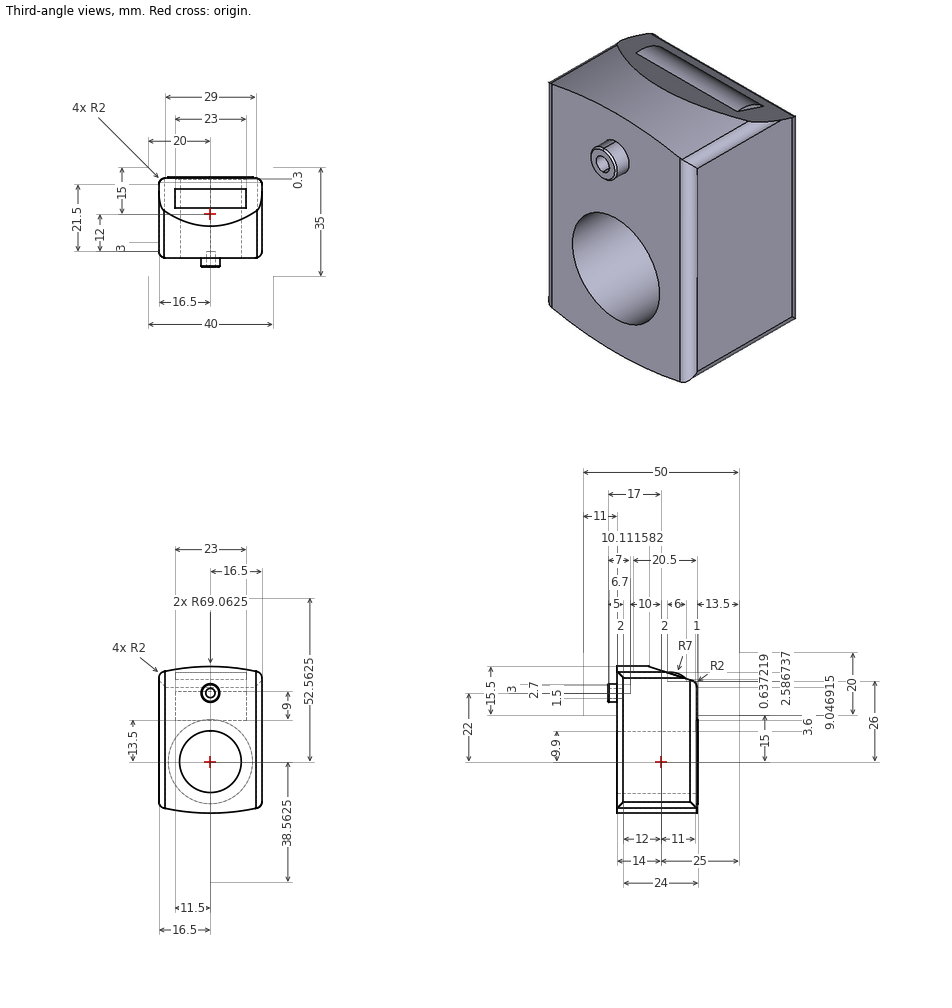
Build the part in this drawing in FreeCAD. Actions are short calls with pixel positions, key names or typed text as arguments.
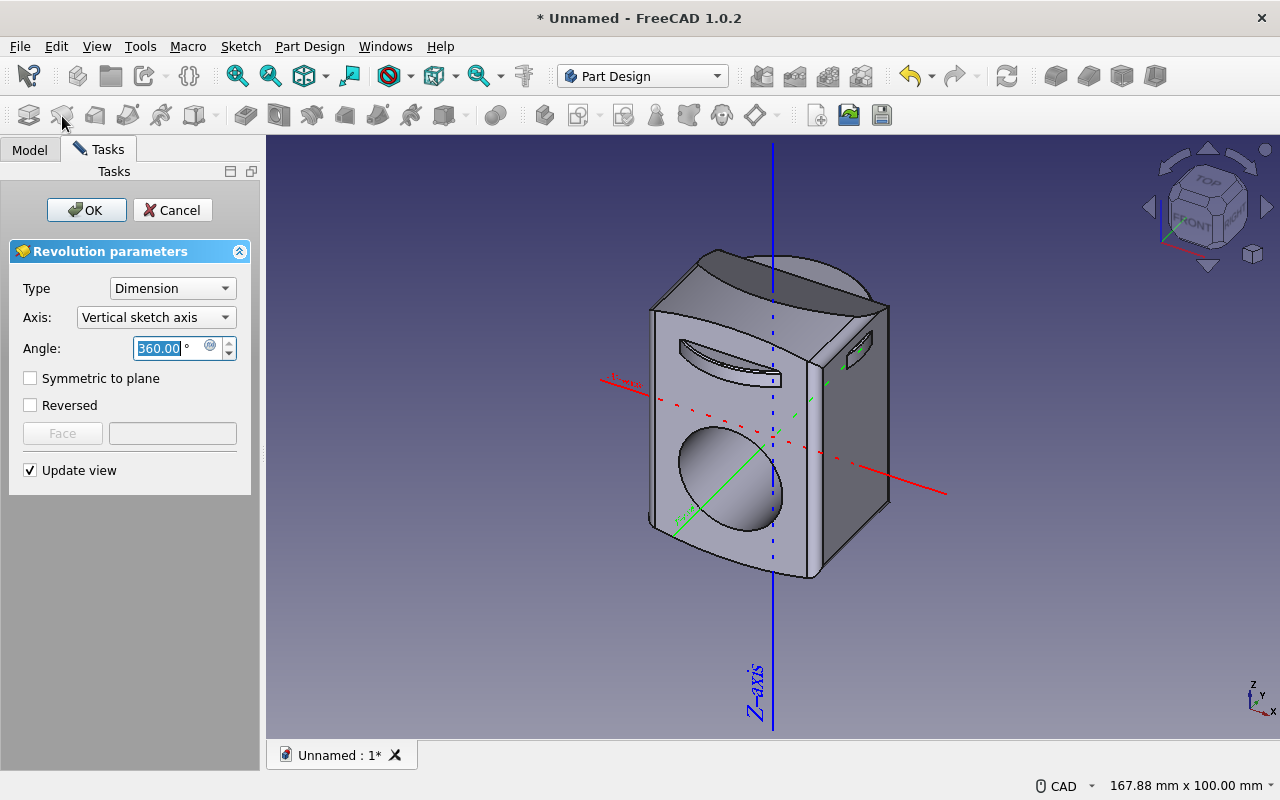
click(157, 318)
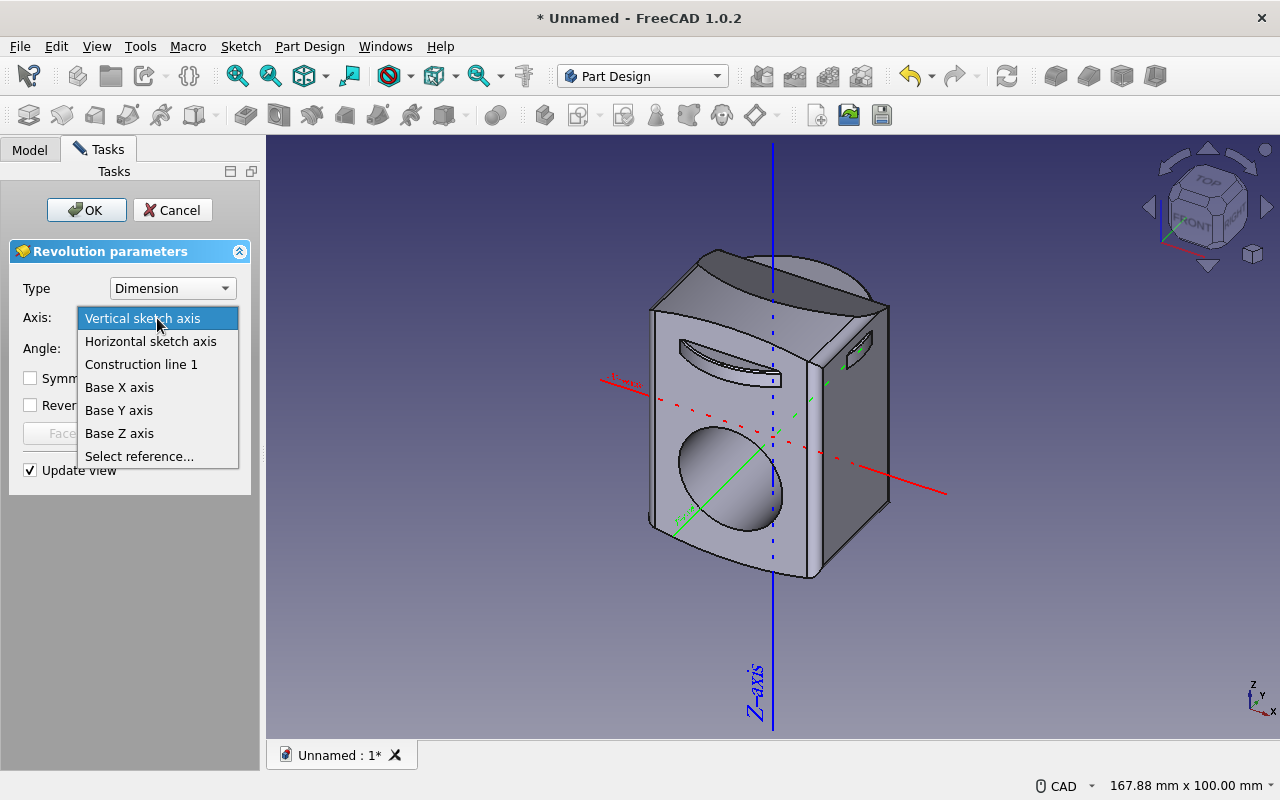
click(156, 364)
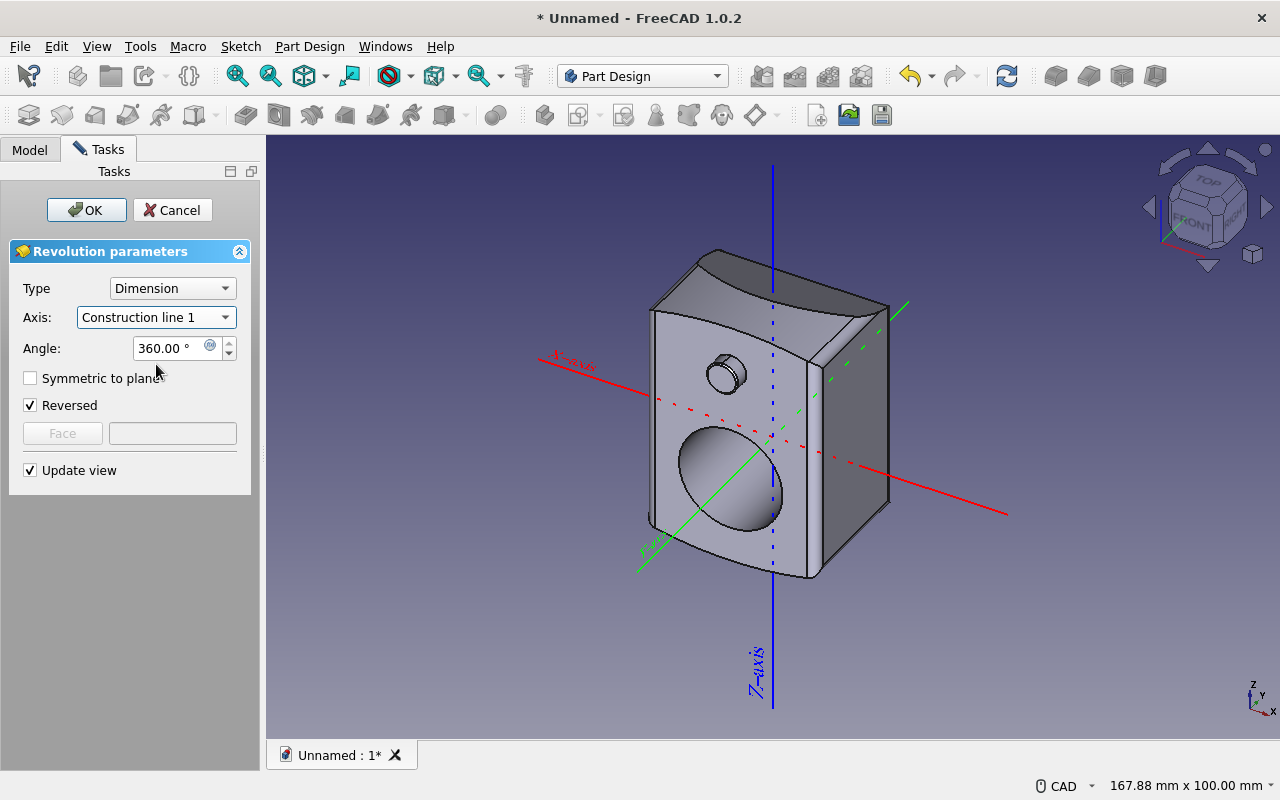
click(87, 210)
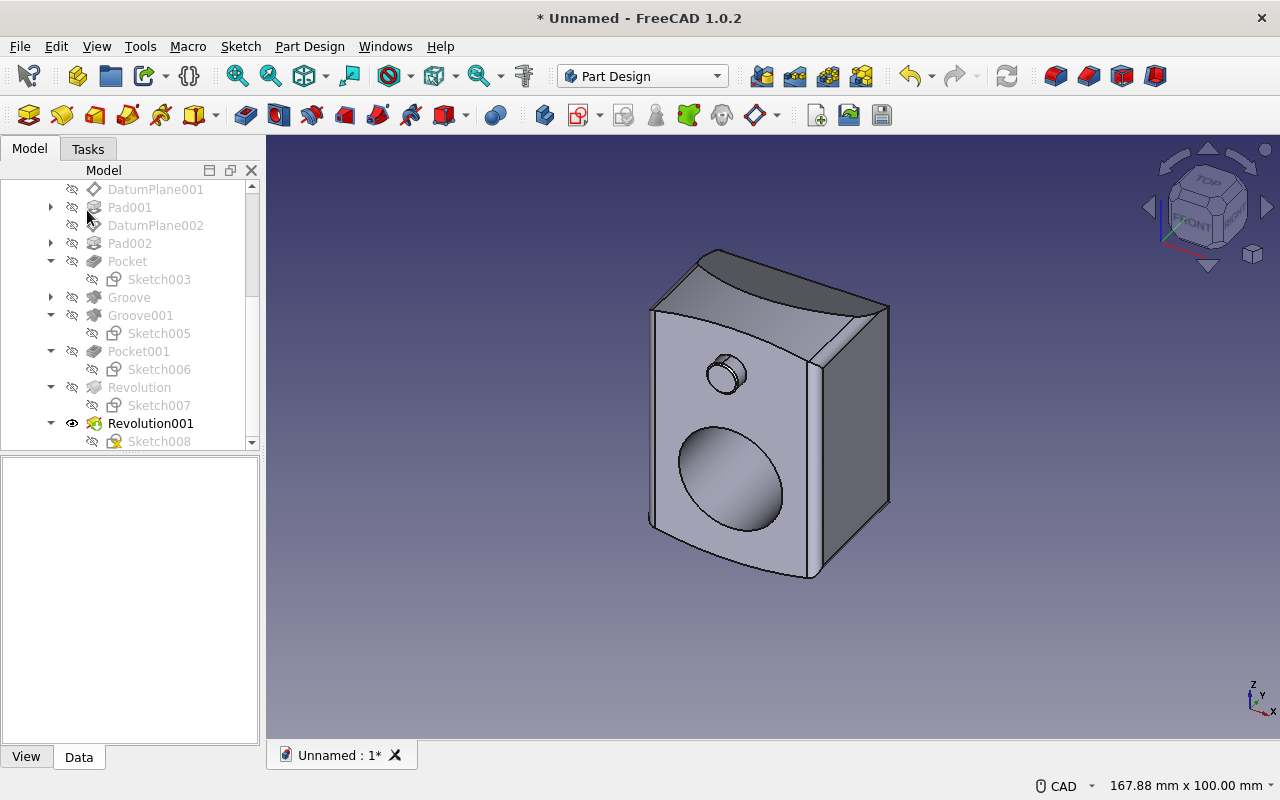
click(578, 116)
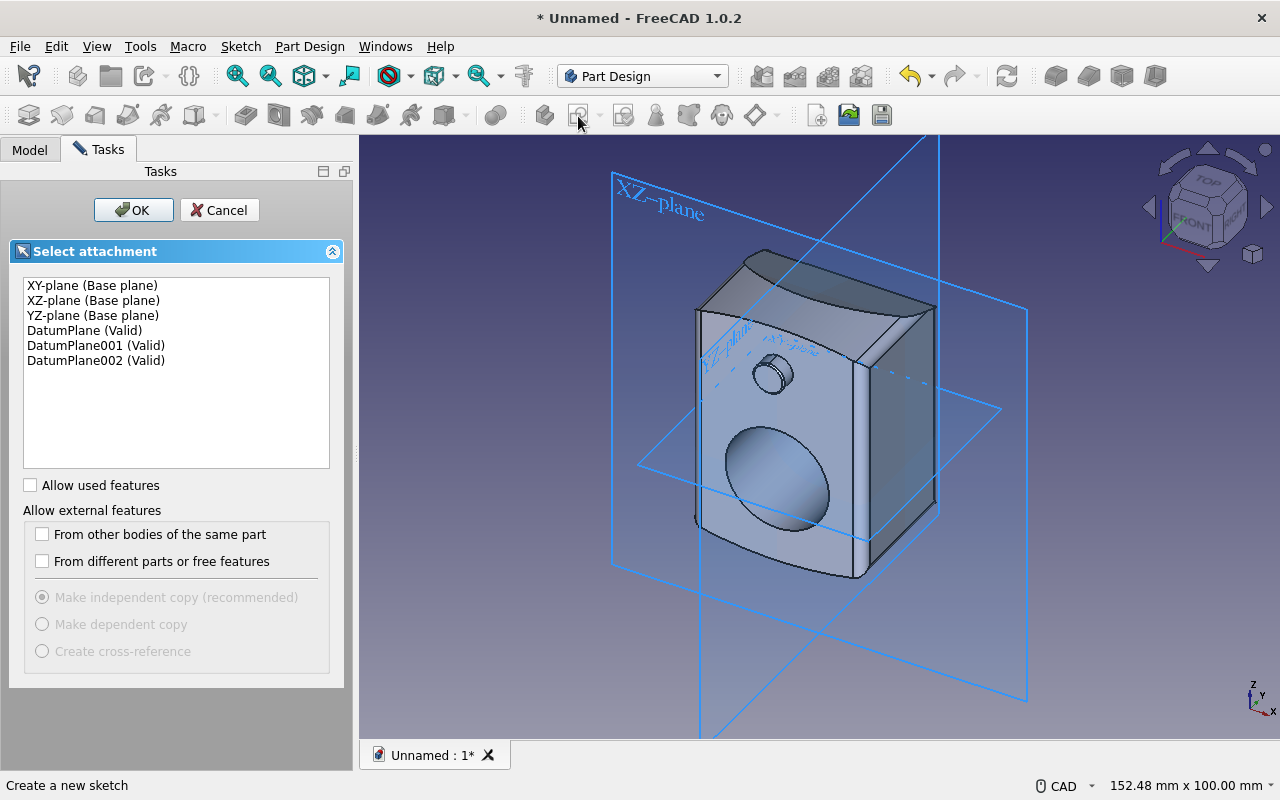
click(84, 316)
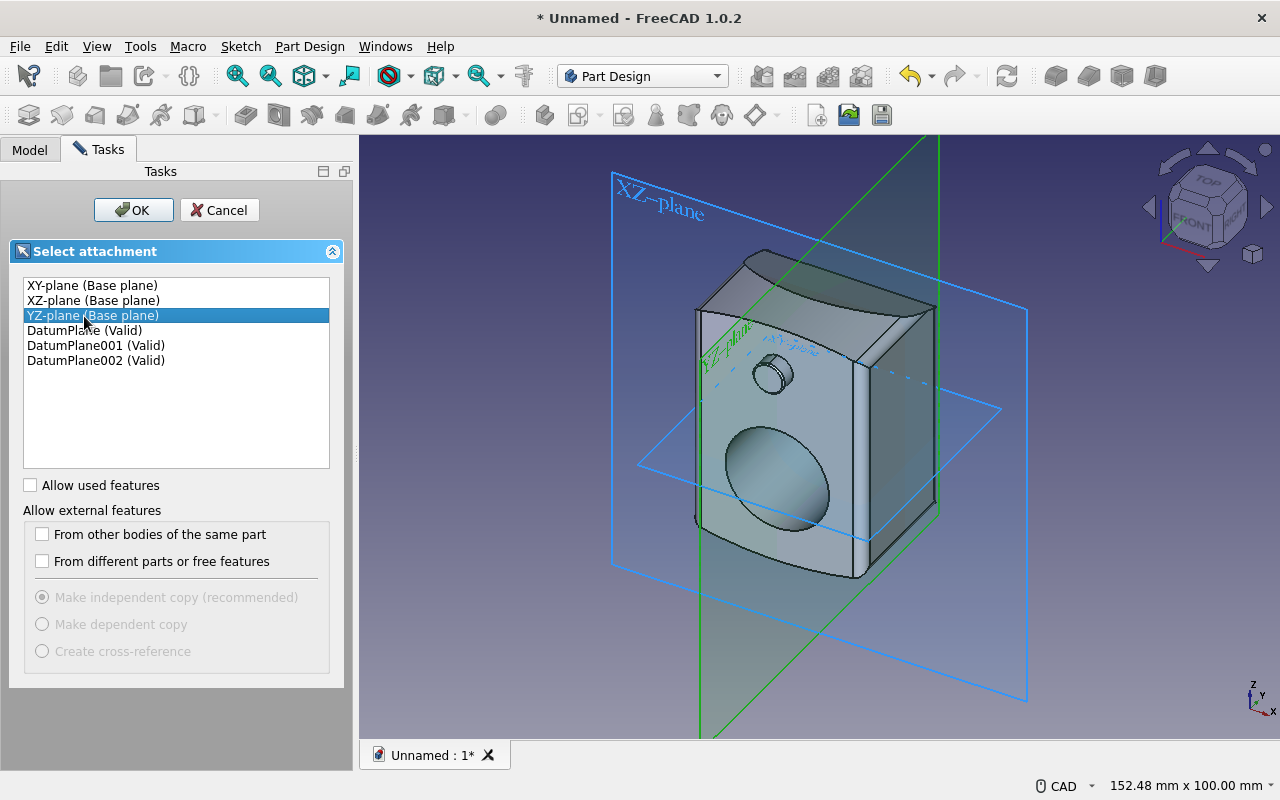
click(134, 210)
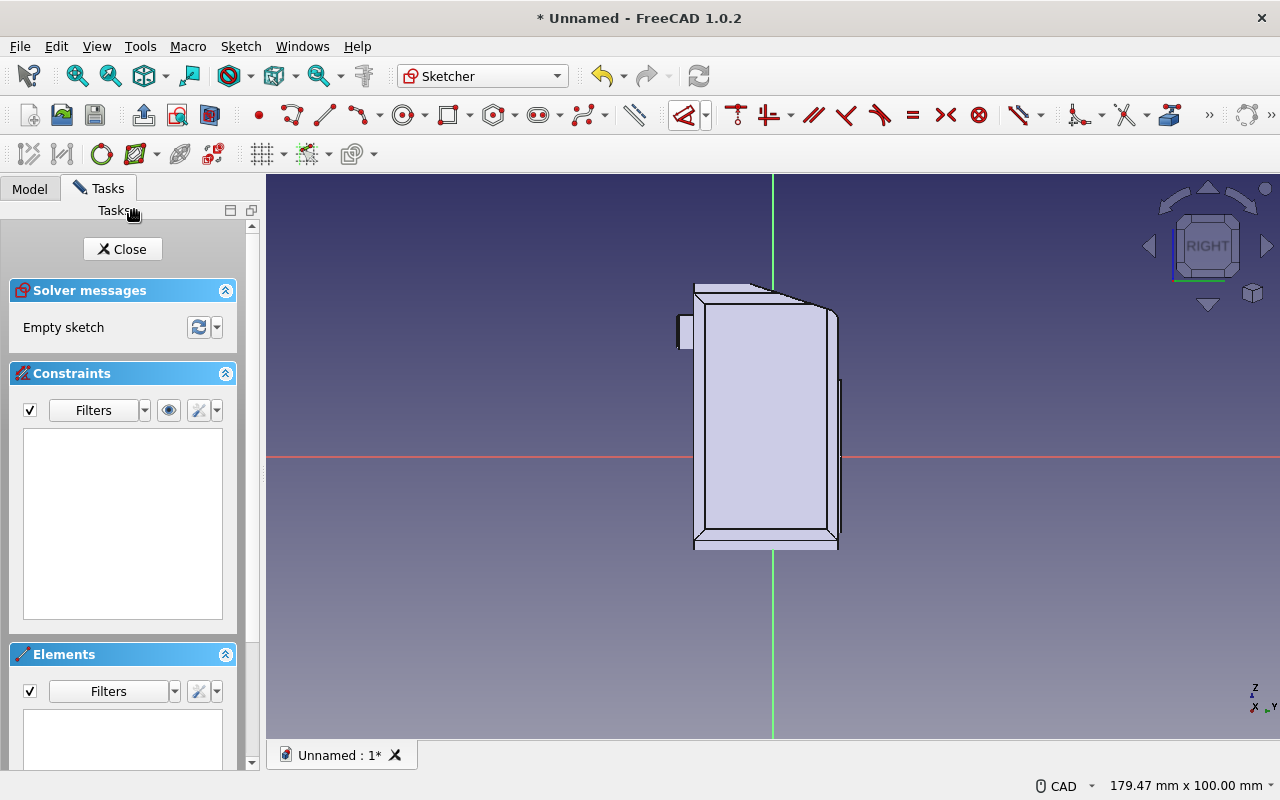
click(210, 116)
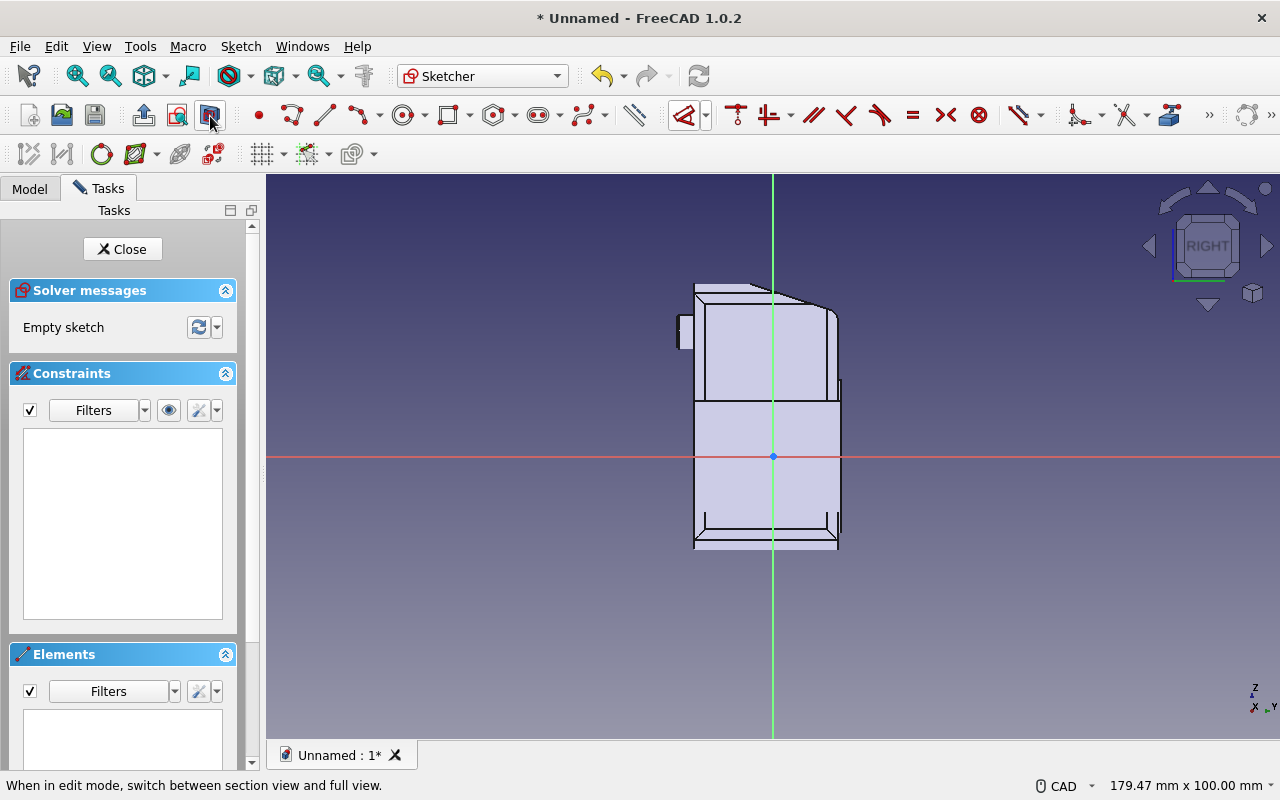
scroll(696, 327, up, 13)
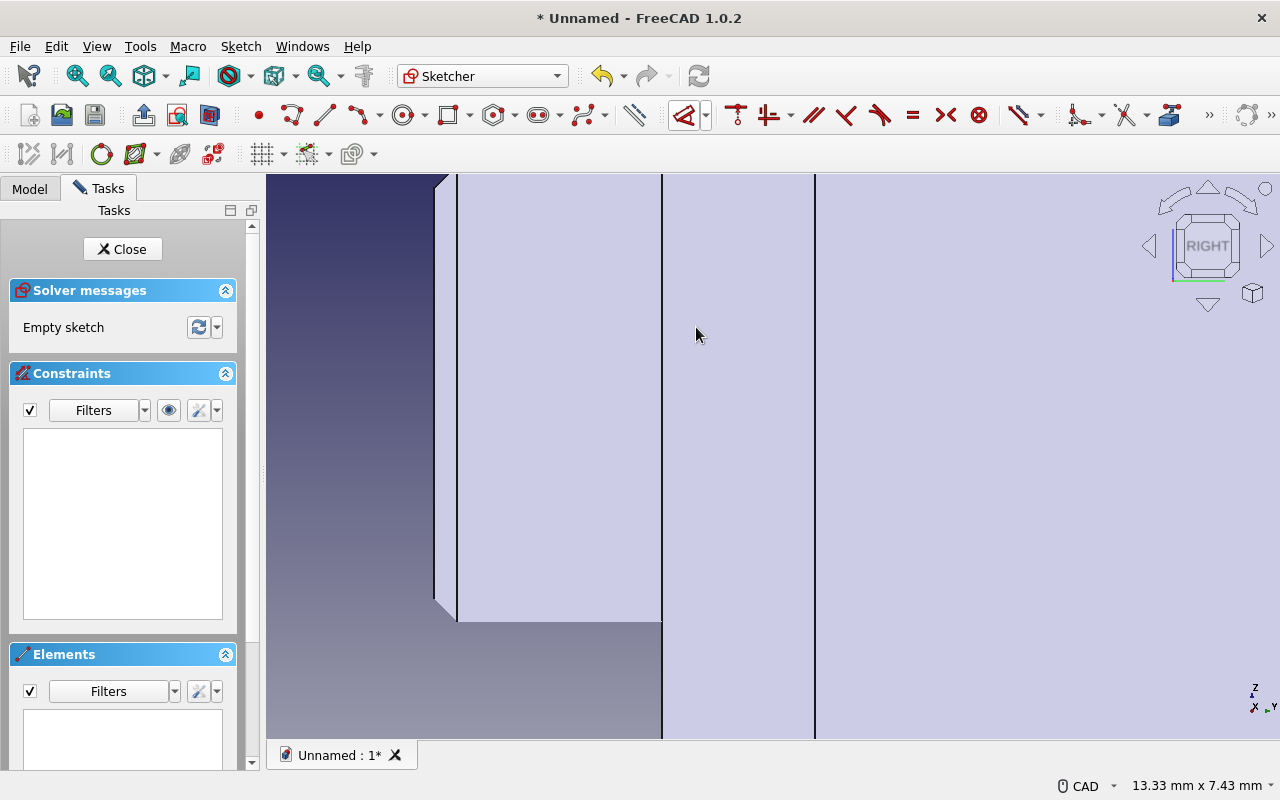
click(448, 116)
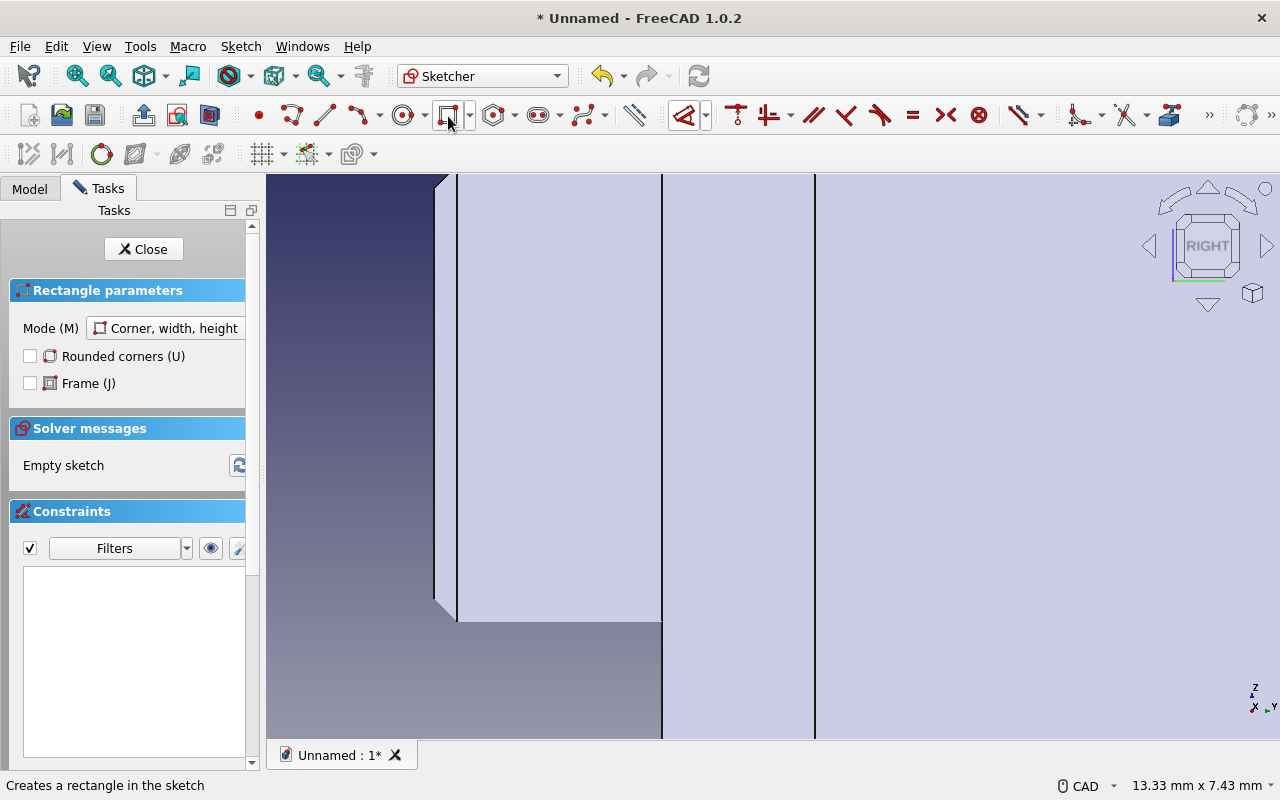
click(434, 394)
move(815, 508)